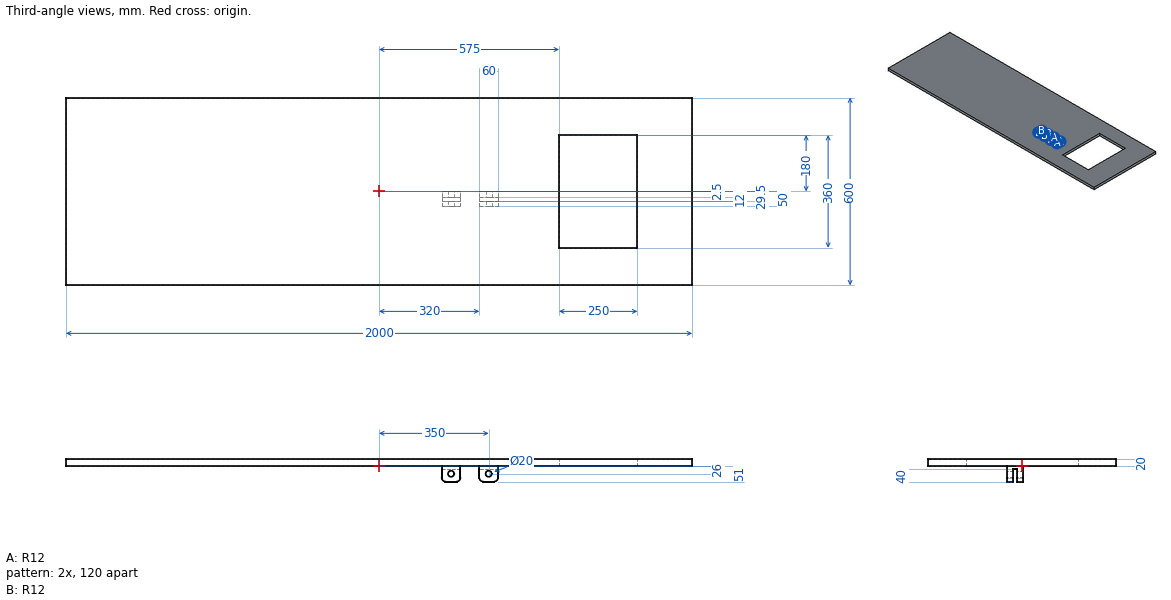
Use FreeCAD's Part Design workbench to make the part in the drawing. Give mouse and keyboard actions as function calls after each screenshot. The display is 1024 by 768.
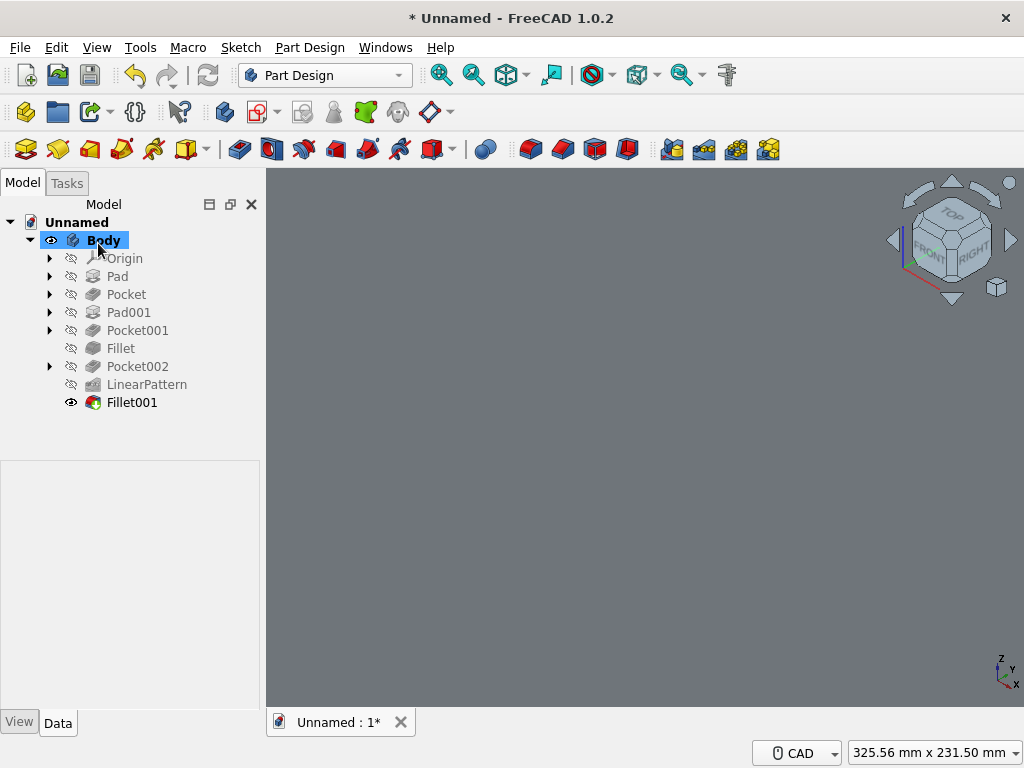
key(v)
key(f)